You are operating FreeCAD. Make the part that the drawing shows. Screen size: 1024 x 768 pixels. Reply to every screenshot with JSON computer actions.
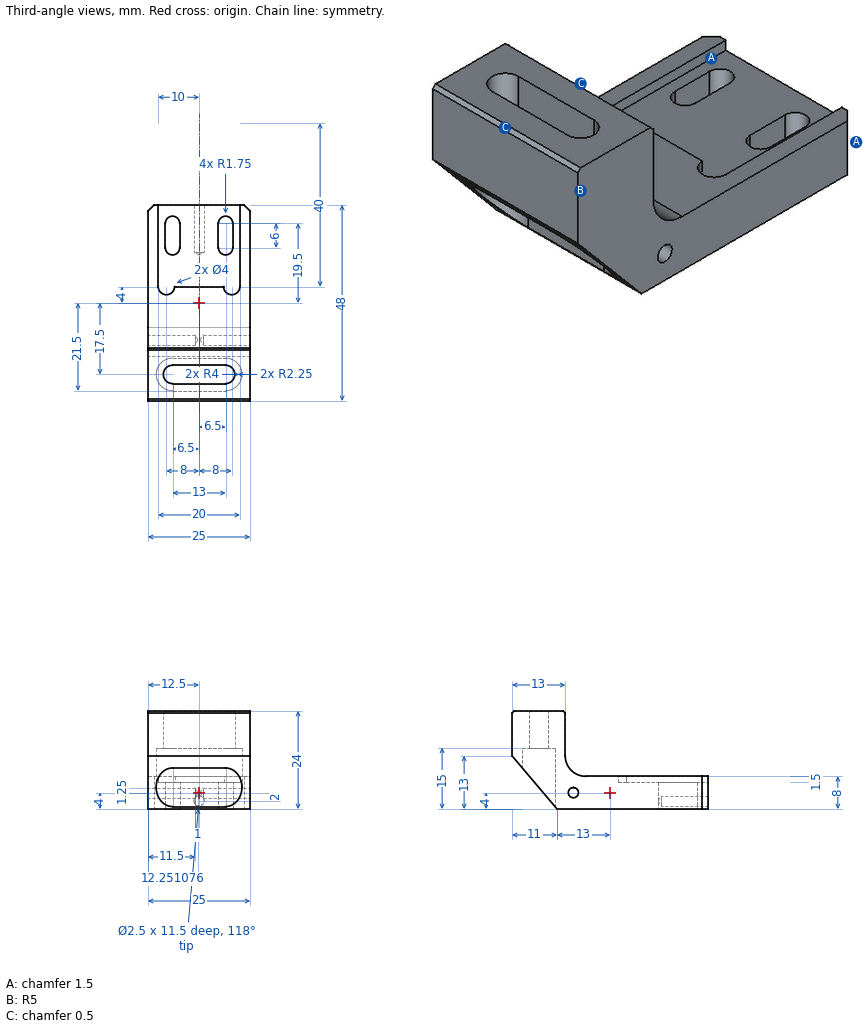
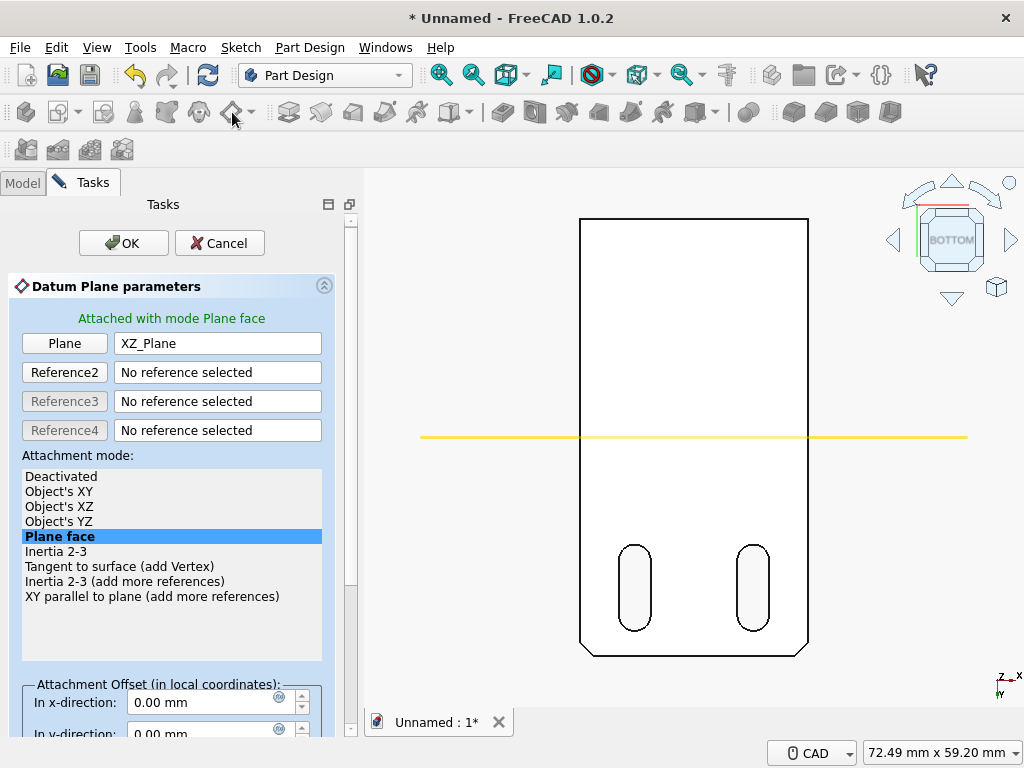
{"action": "scroll", "coordinate": [351, 475], "scroll_direction": "down", "scroll_amount": 2}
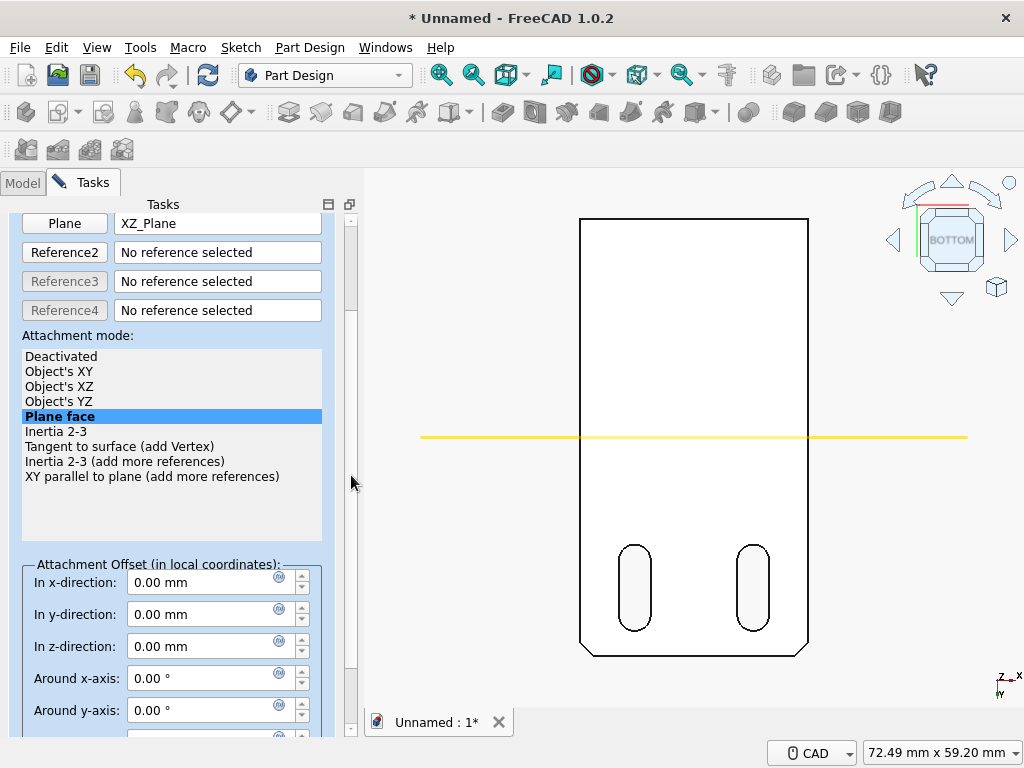
{"action": "triple_click", "coordinate": [210, 646]}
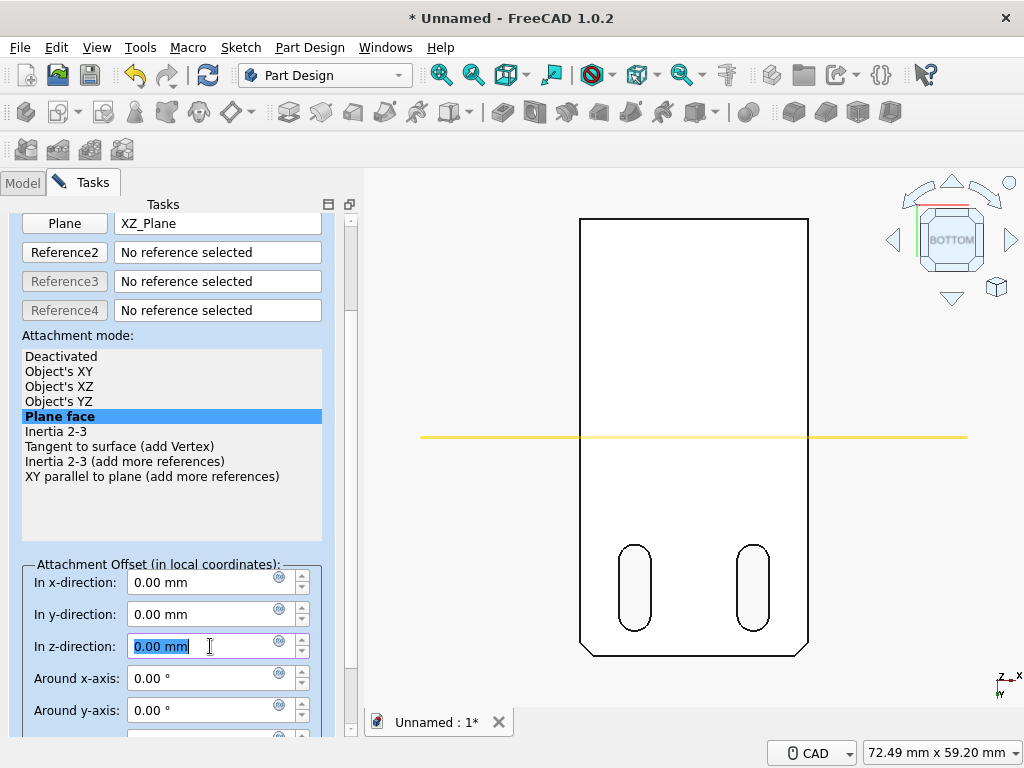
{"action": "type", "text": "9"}
{"action": "key", "text": "Tab"}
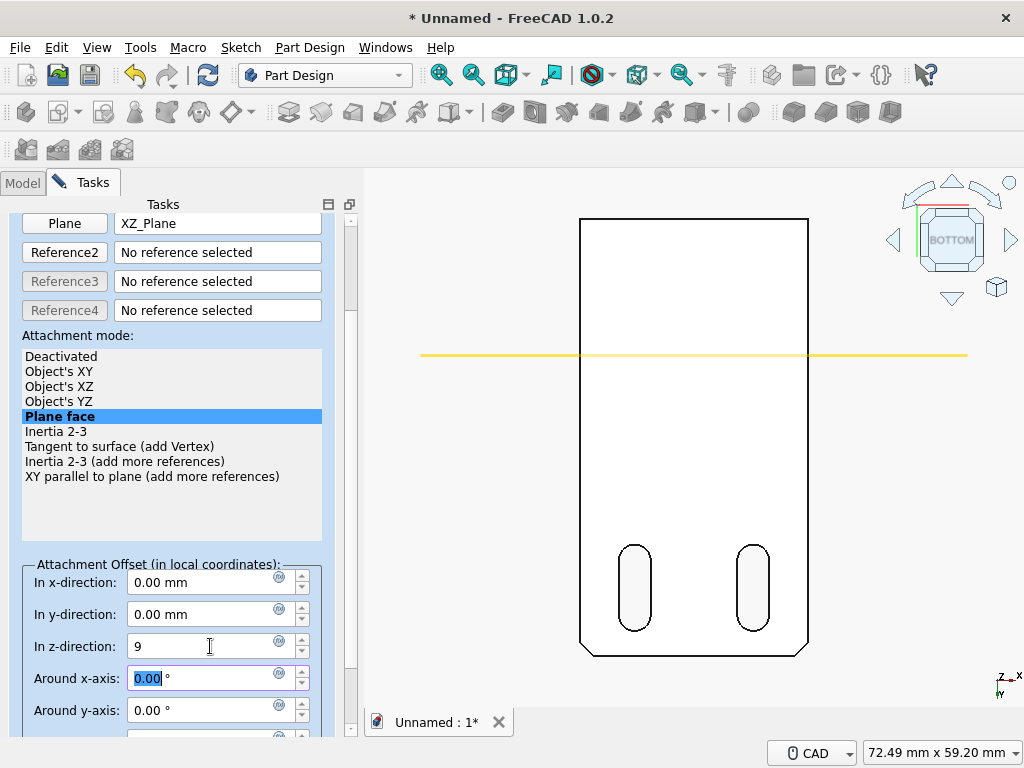
{"action": "scroll", "coordinate": [351, 475], "scroll_direction": "up", "scroll_amount": 3}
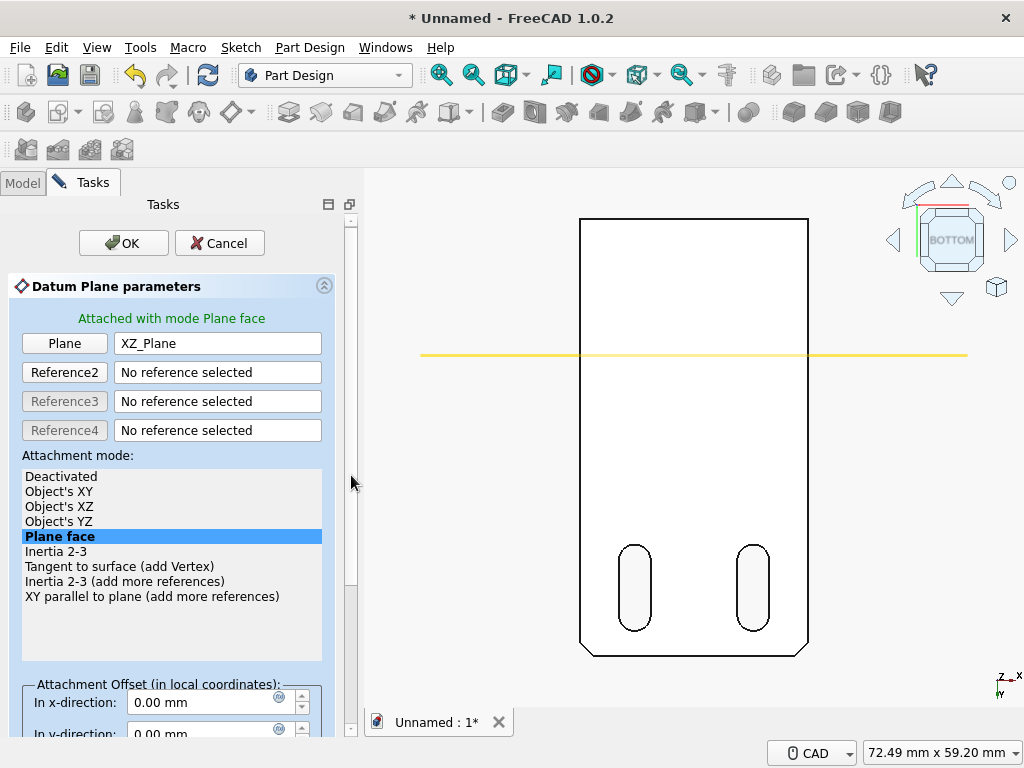
{"action": "left_click", "coordinate": [124, 243]}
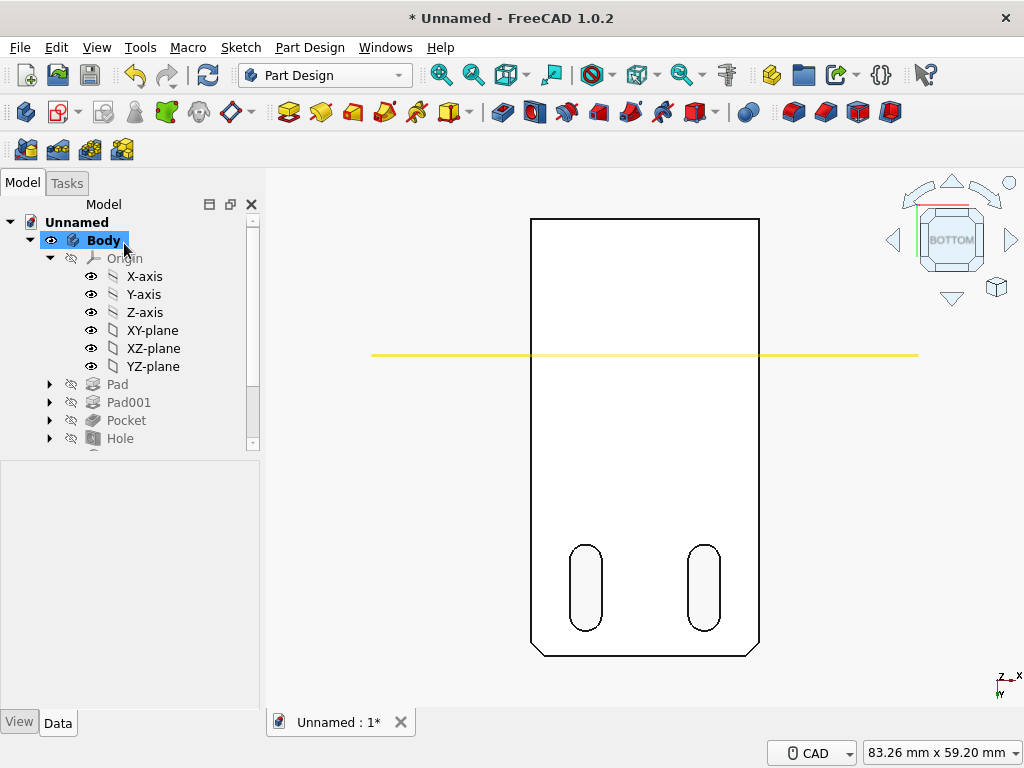
{"action": "scroll", "coordinate": [100, 326], "scroll_direction": "down", "scroll_amount": 3}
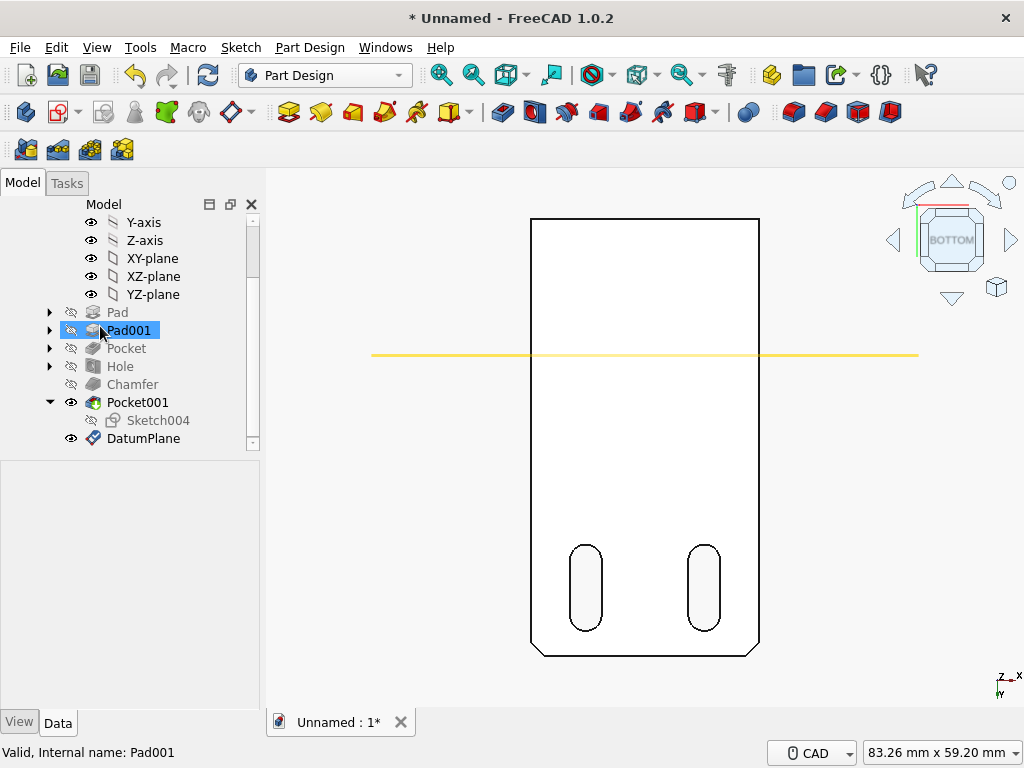
{"action": "left_click", "coordinate": [116, 438]}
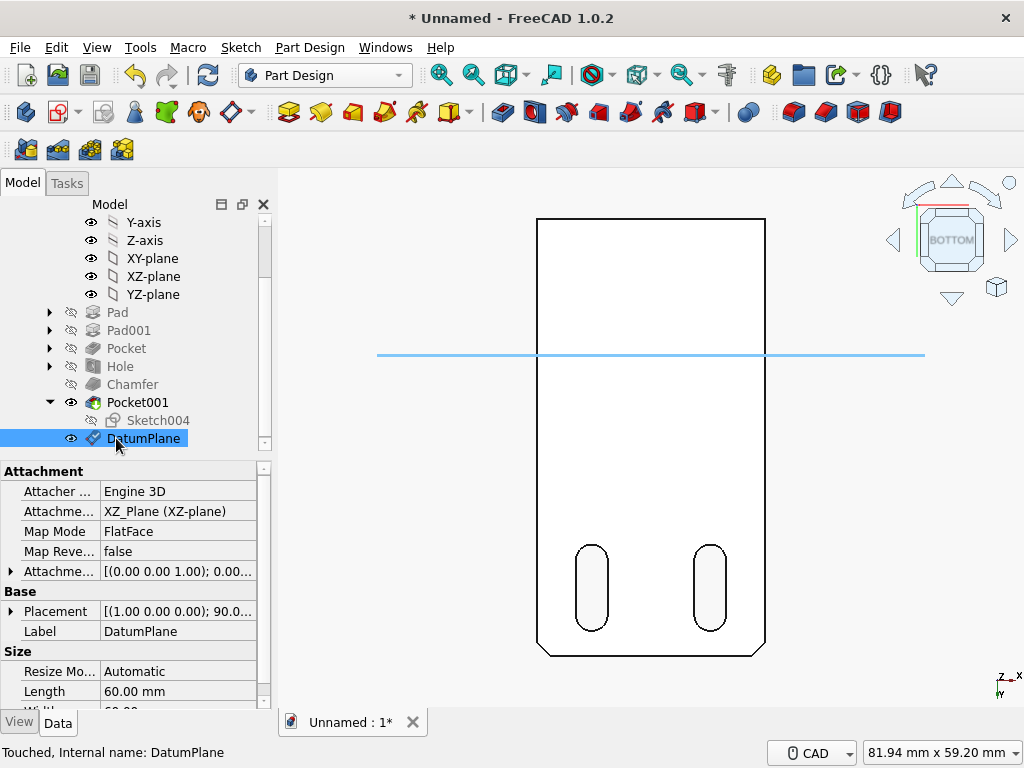
{"action": "left_click", "coordinate": [58, 112]}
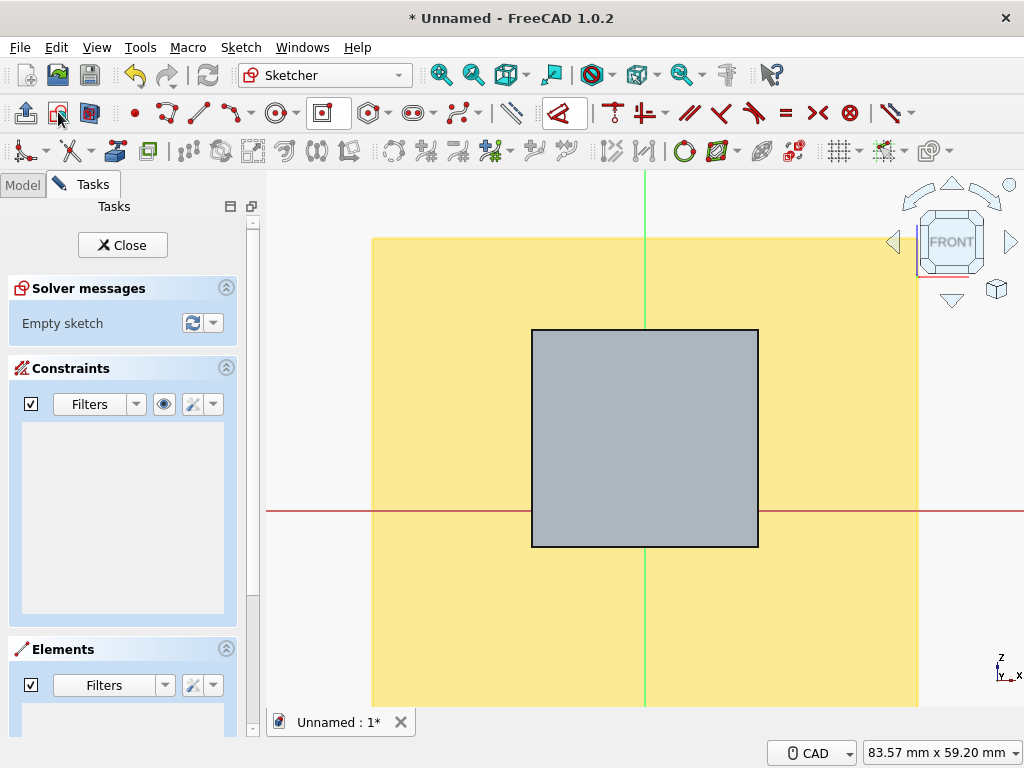
{"action": "left_click", "coordinate": [90, 114]}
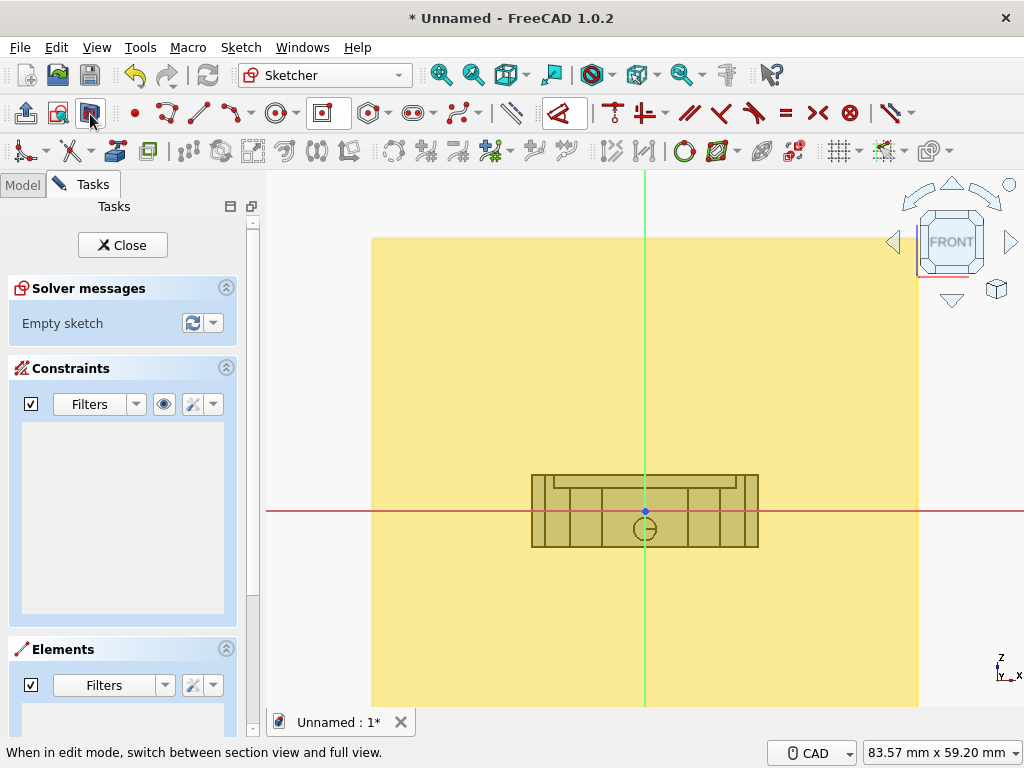
{"action": "scroll", "coordinate": [593, 534], "scroll_direction": "up", "scroll_amount": 6}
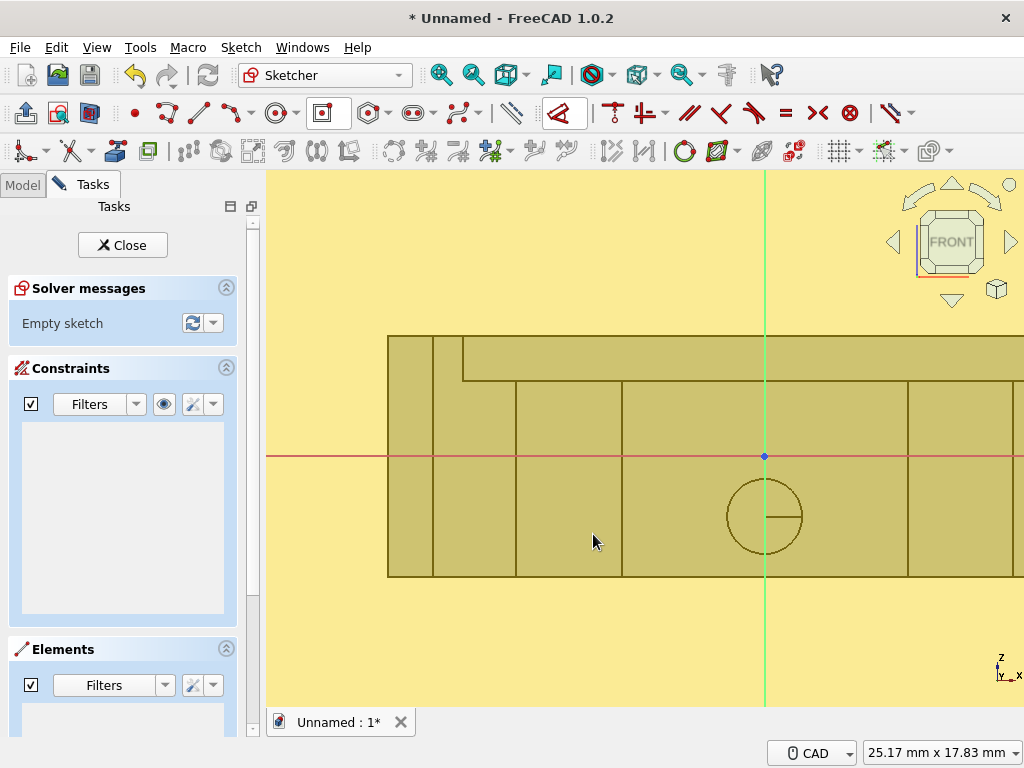
{"action": "left_click", "coordinate": [168, 114]}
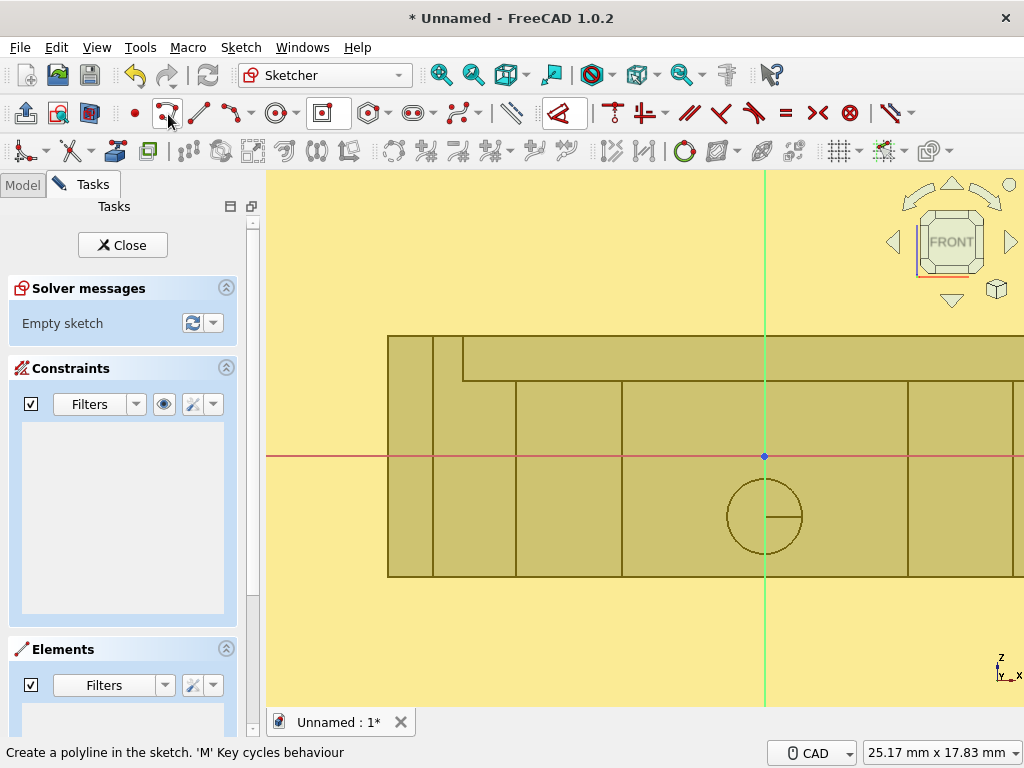
{"action": "scroll", "coordinate": [757, 456], "scroll_direction": "up", "scroll_amount": 4}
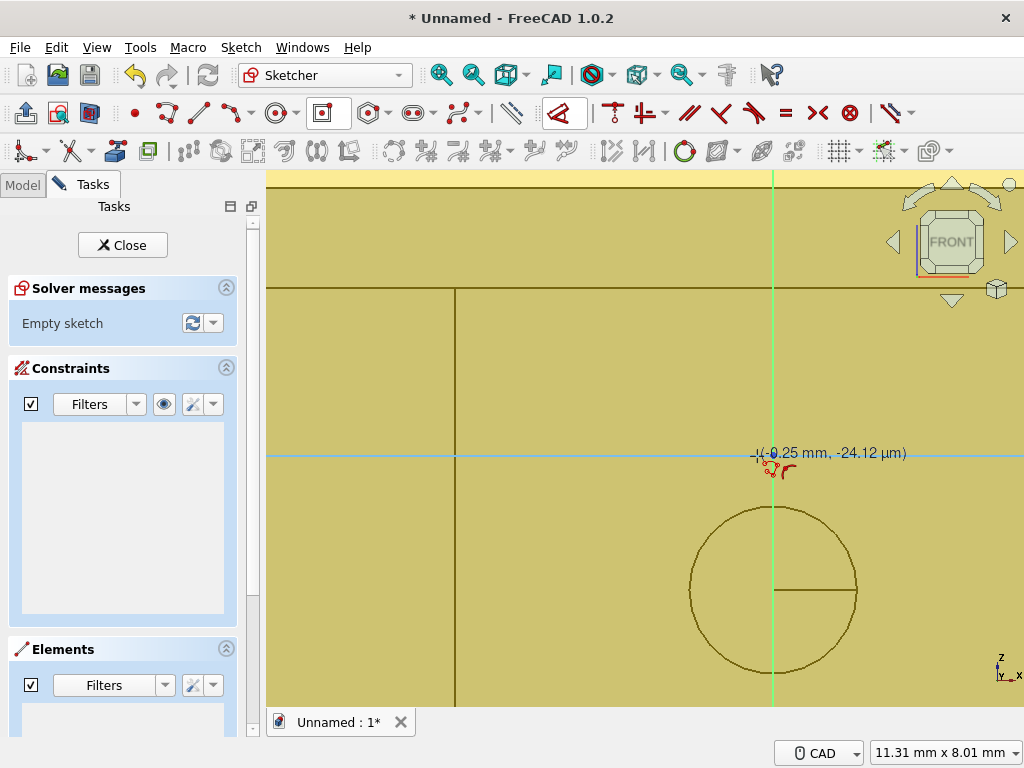
{"action": "left_click", "coordinate": [757, 456]}